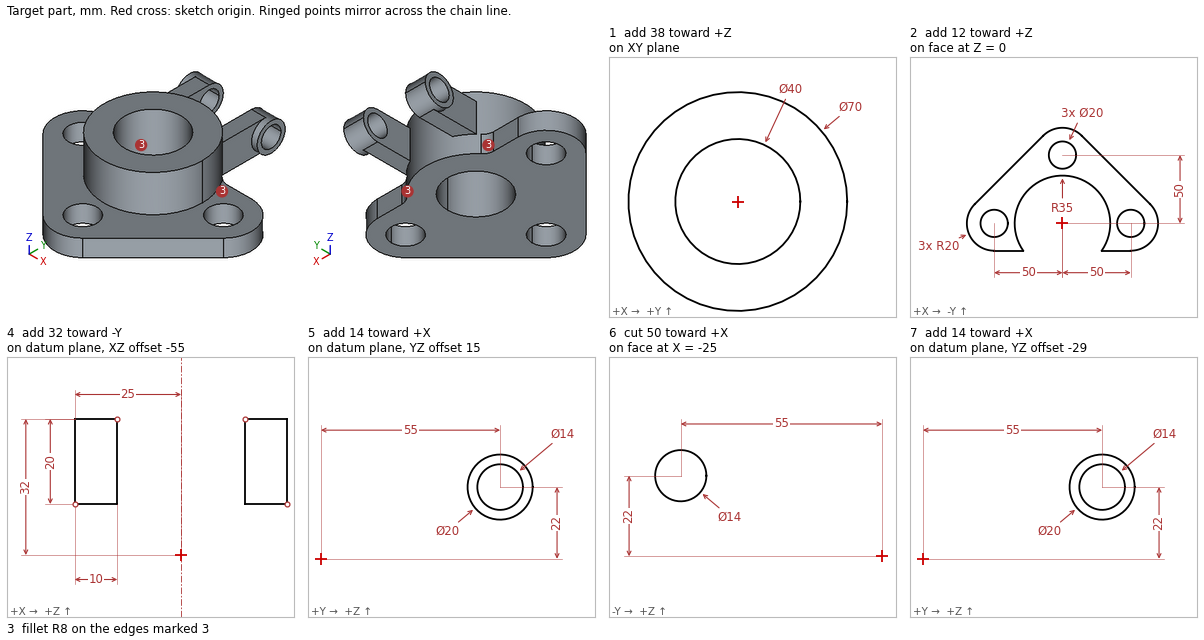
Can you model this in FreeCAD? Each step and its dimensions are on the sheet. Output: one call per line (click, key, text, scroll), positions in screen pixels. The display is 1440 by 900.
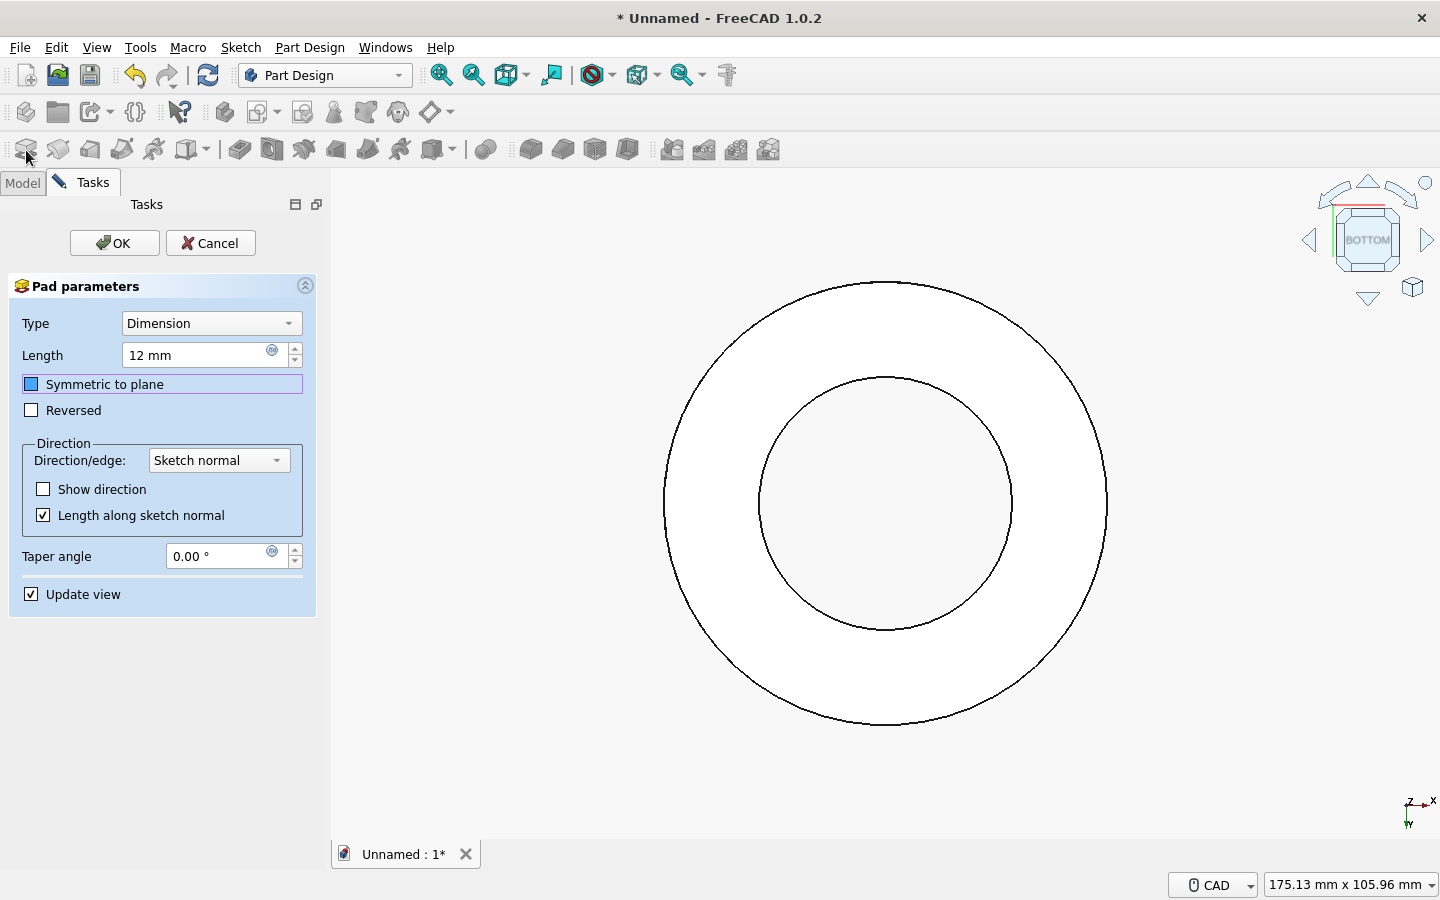
click(30, 410)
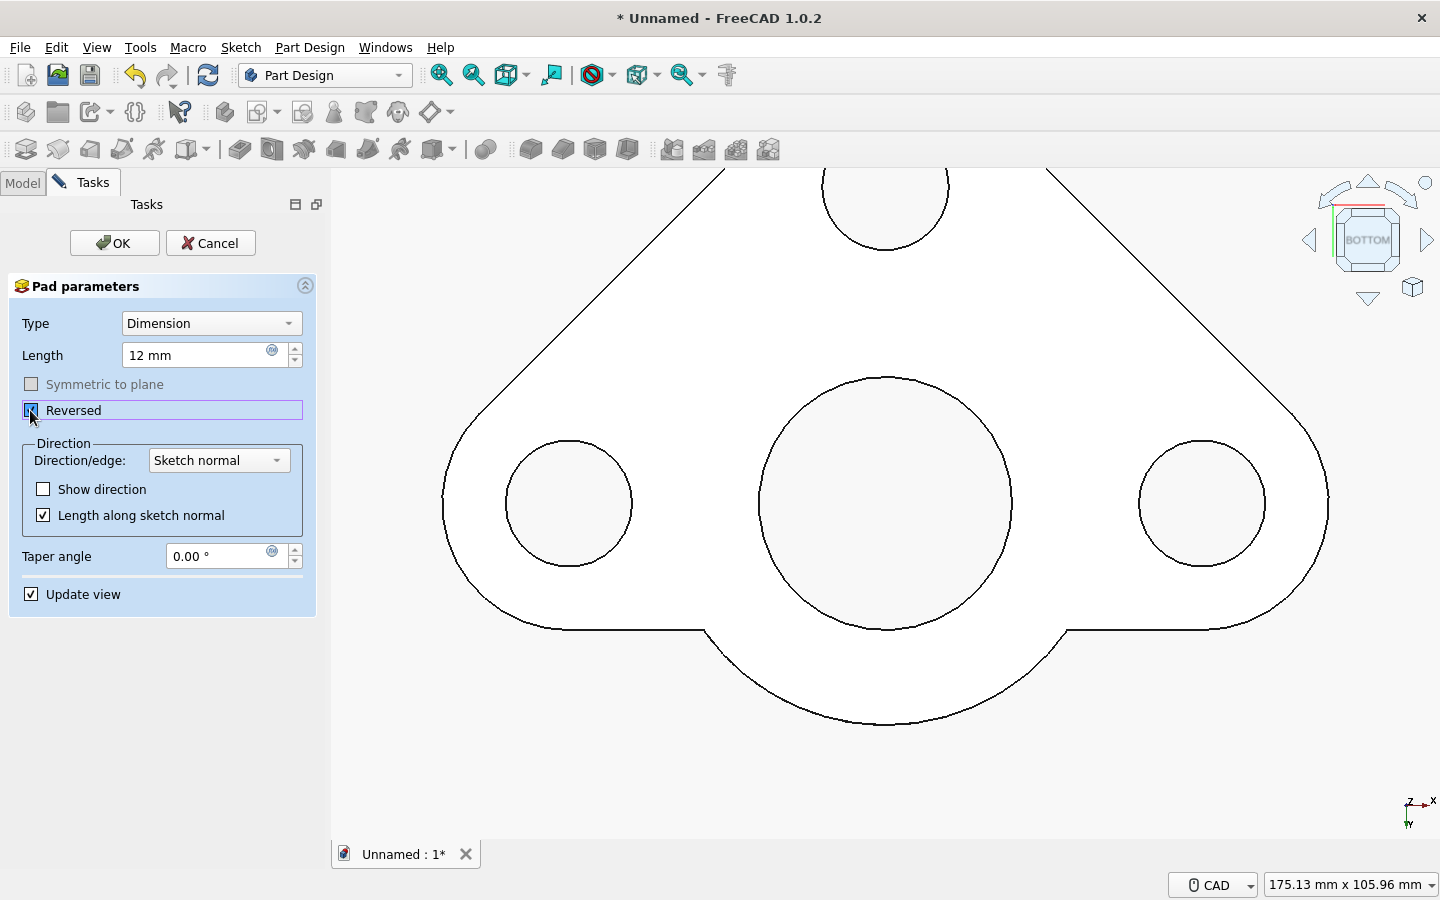
click(115, 243)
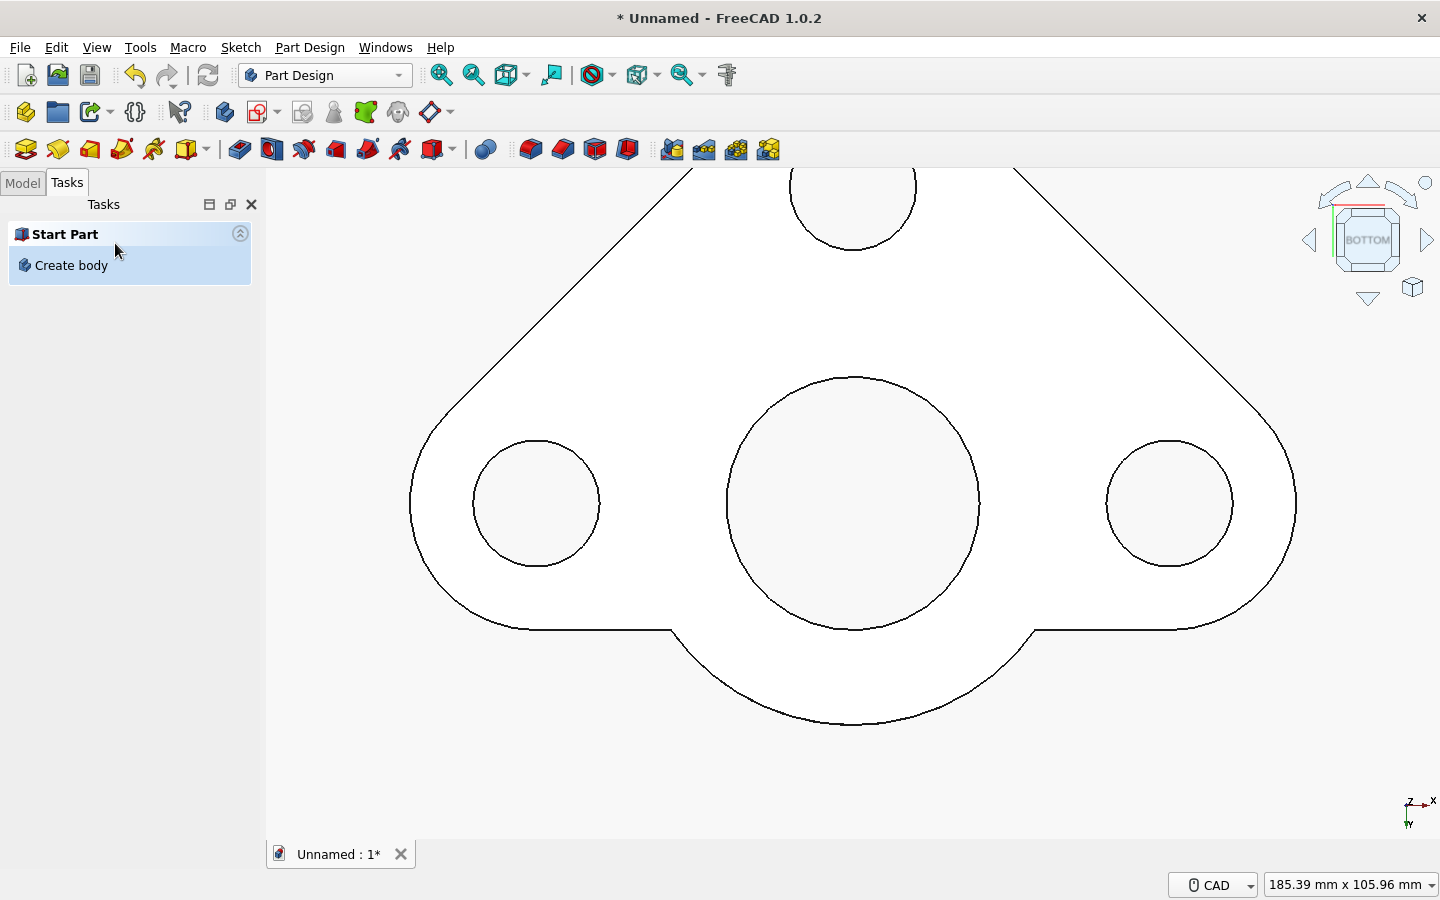
key(v)
key(f)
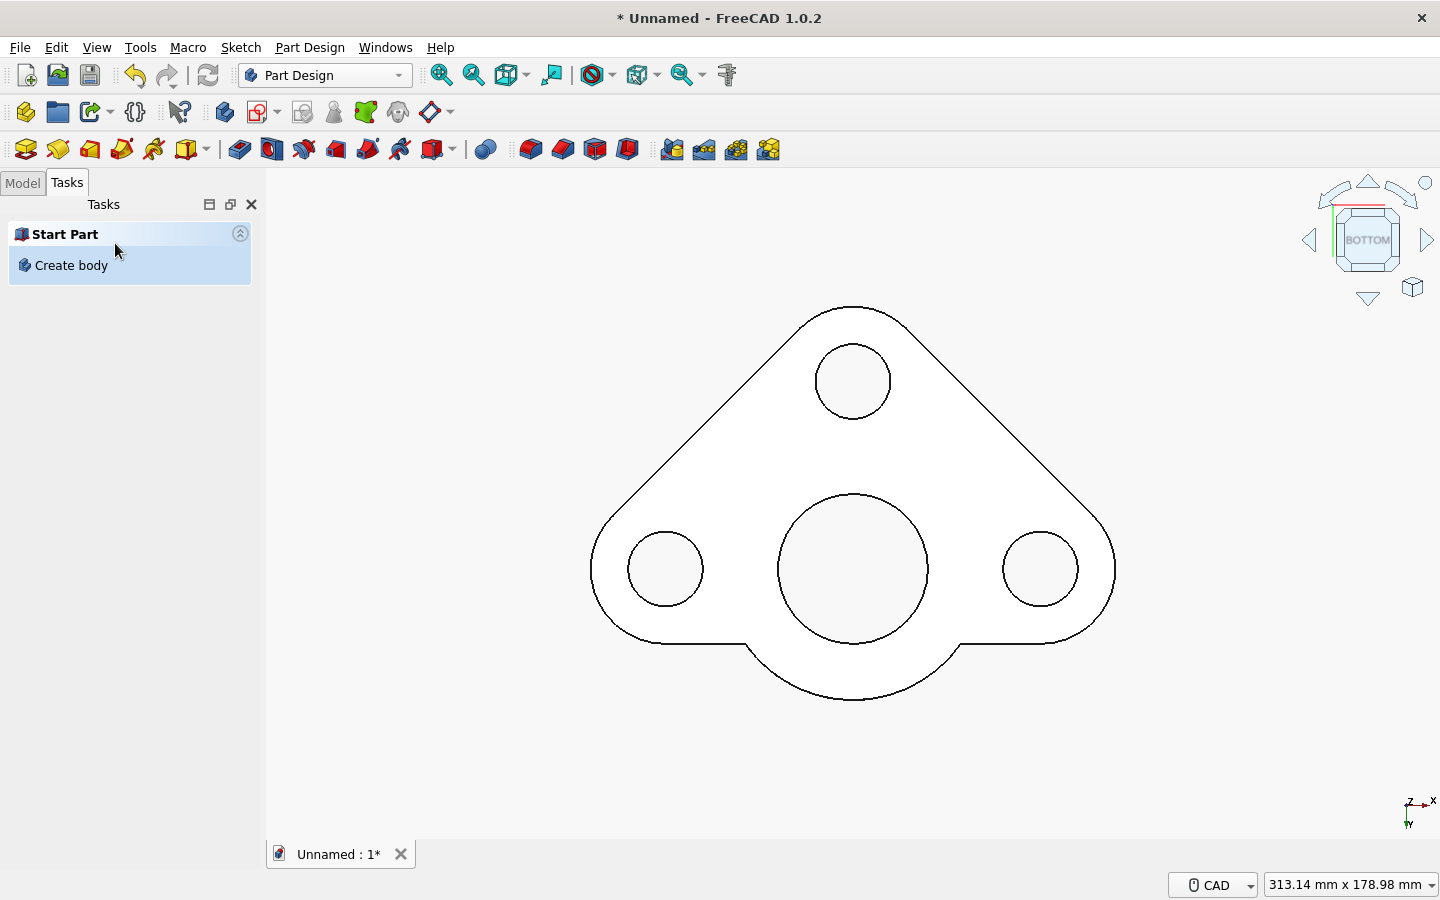
key(0)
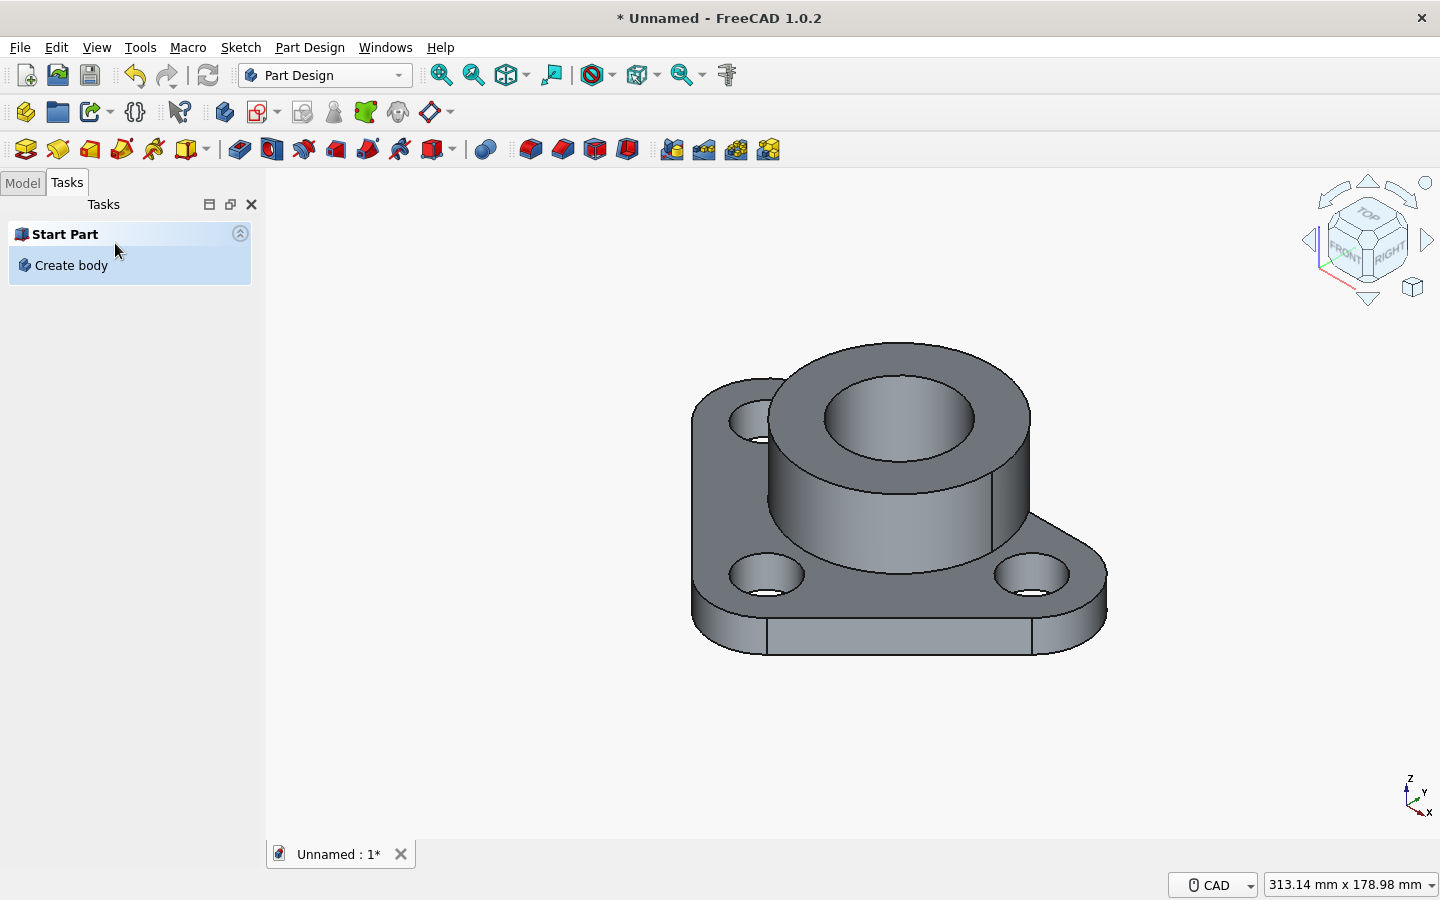
key(2)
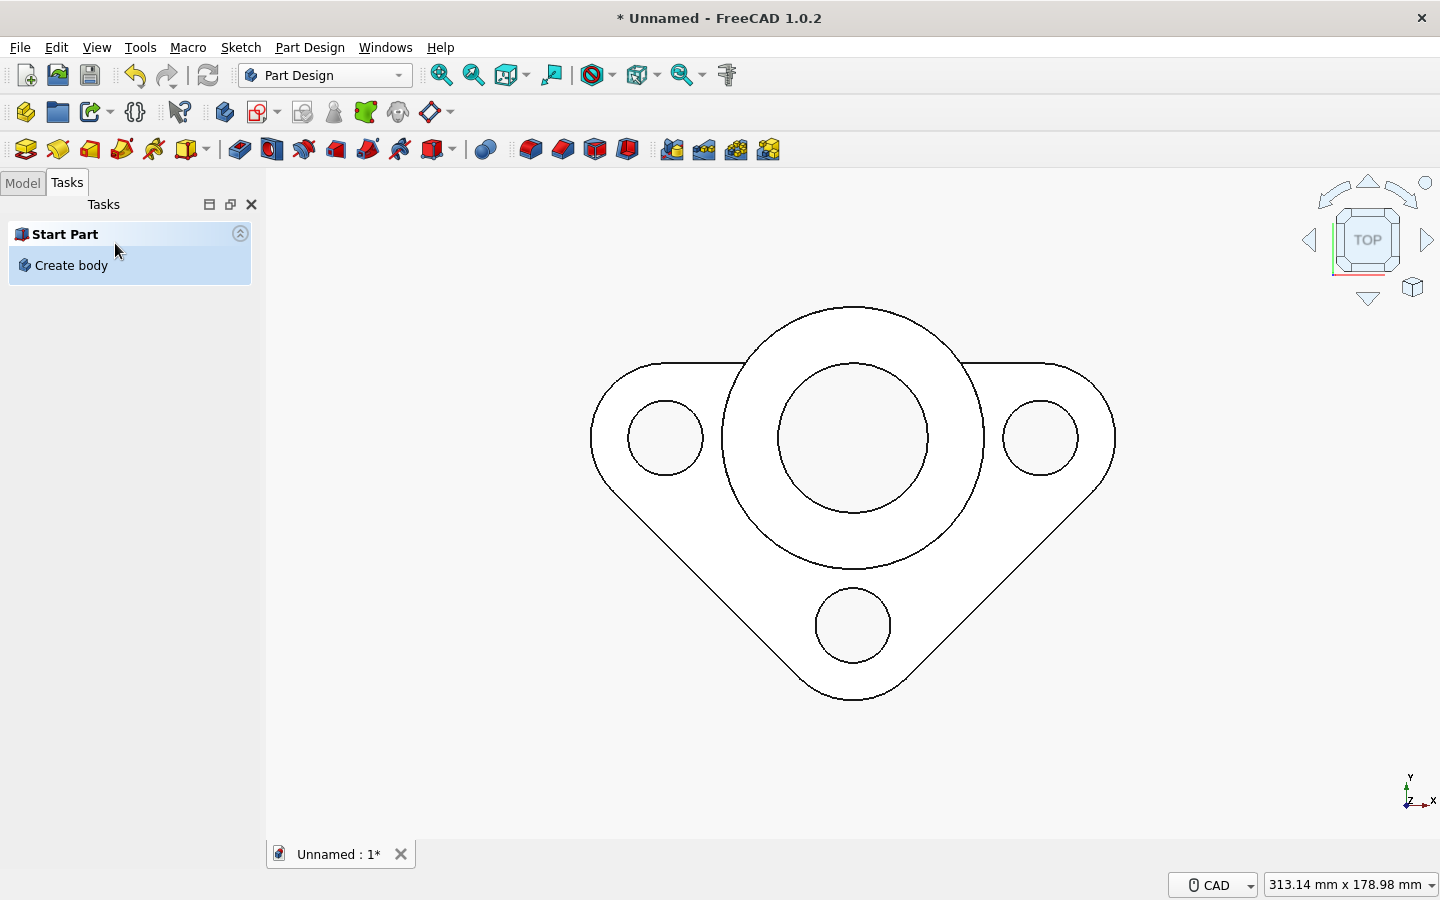
key(1)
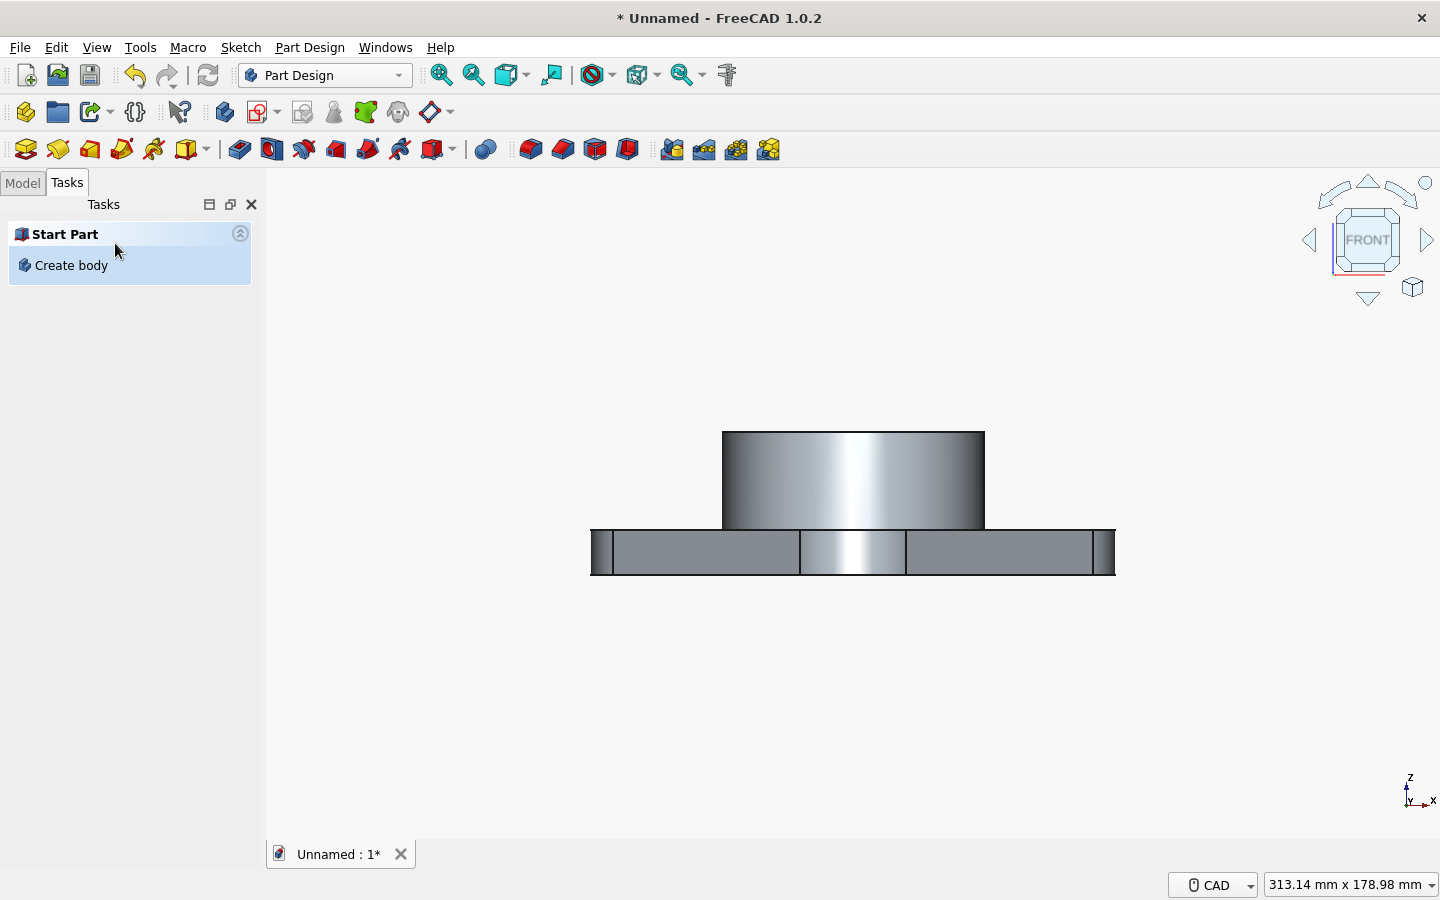
key(v)
key(f)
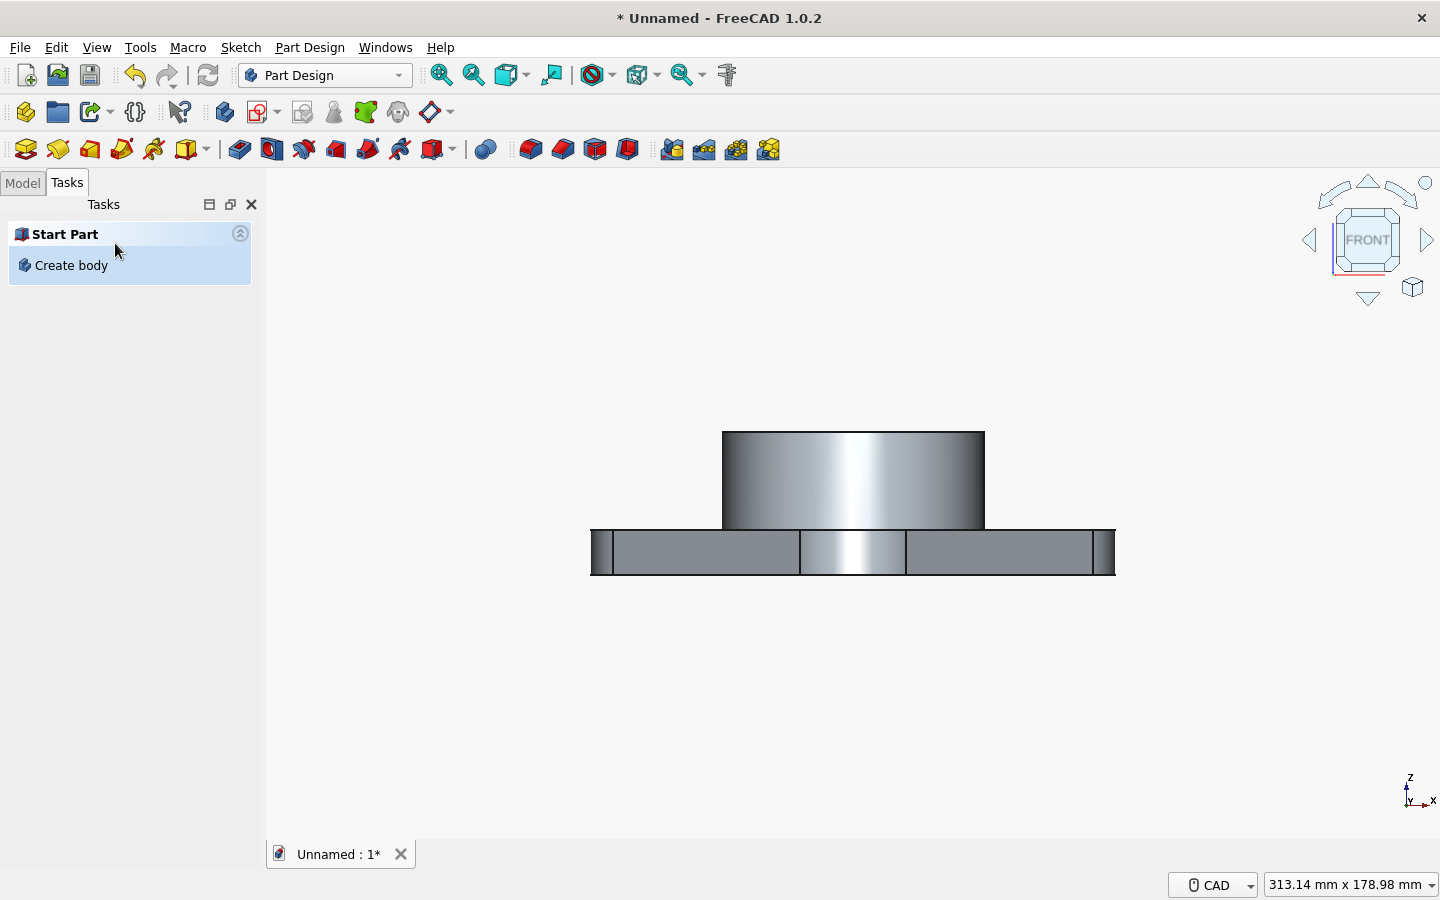
key(3)